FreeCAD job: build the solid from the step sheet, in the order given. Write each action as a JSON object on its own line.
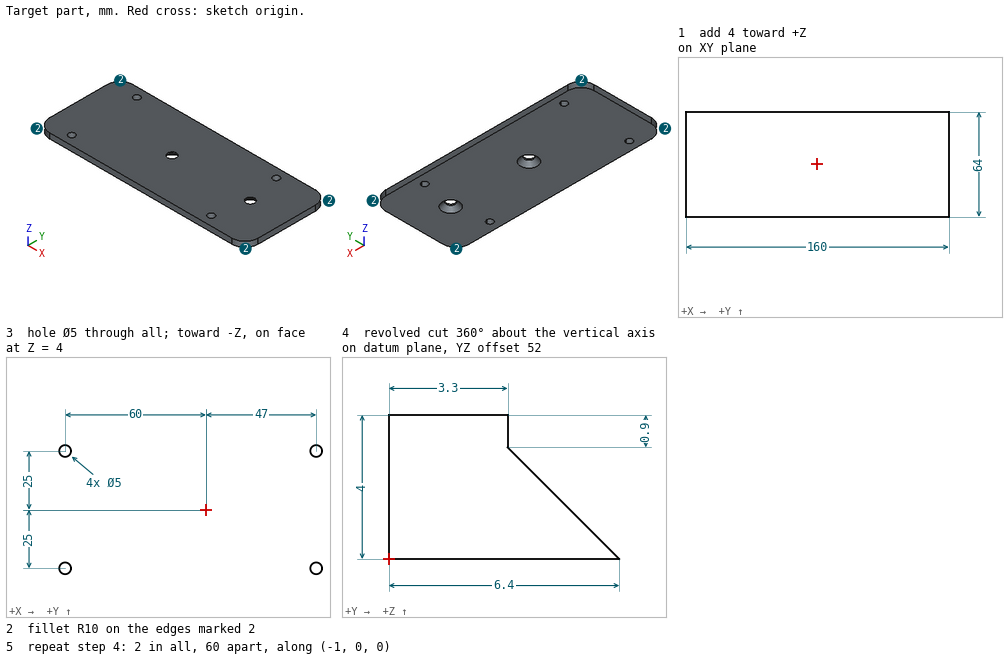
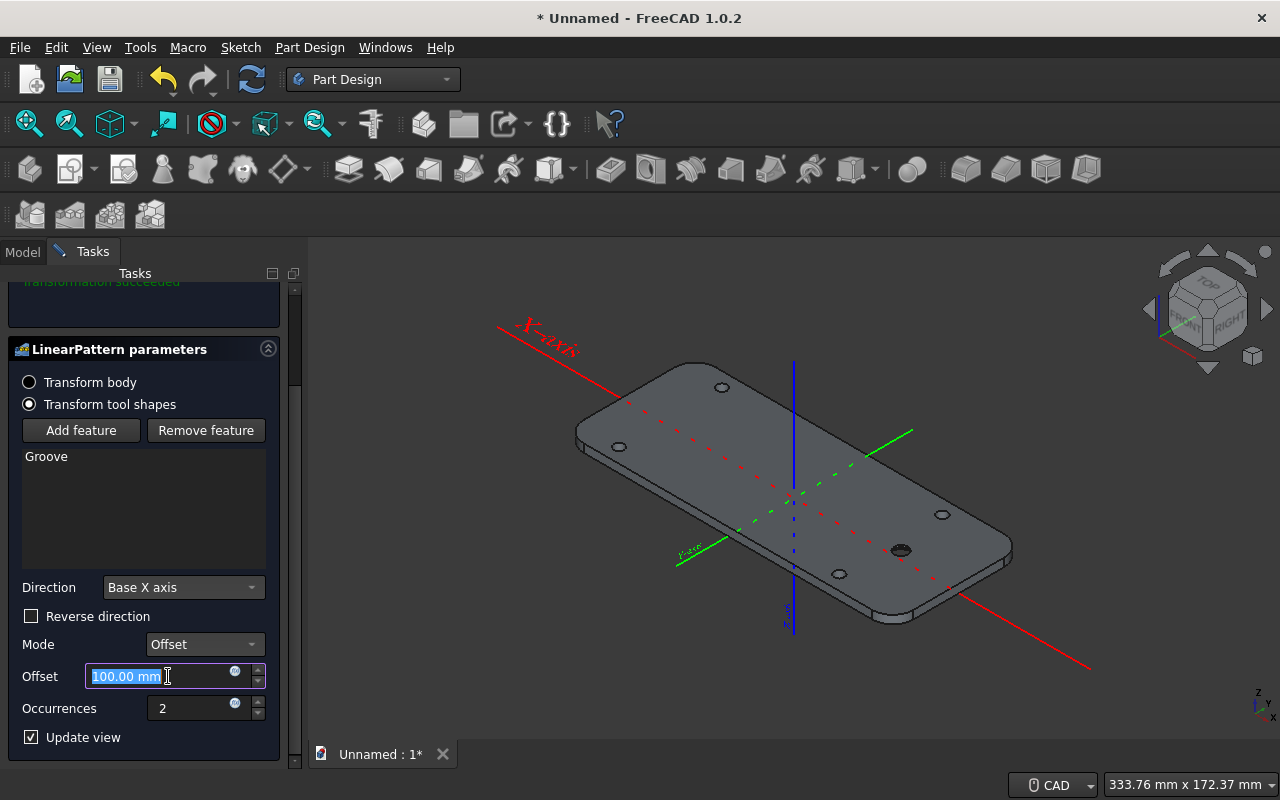
{"action": "type", "text": "60"}
{"action": "key", "text": "Tab"}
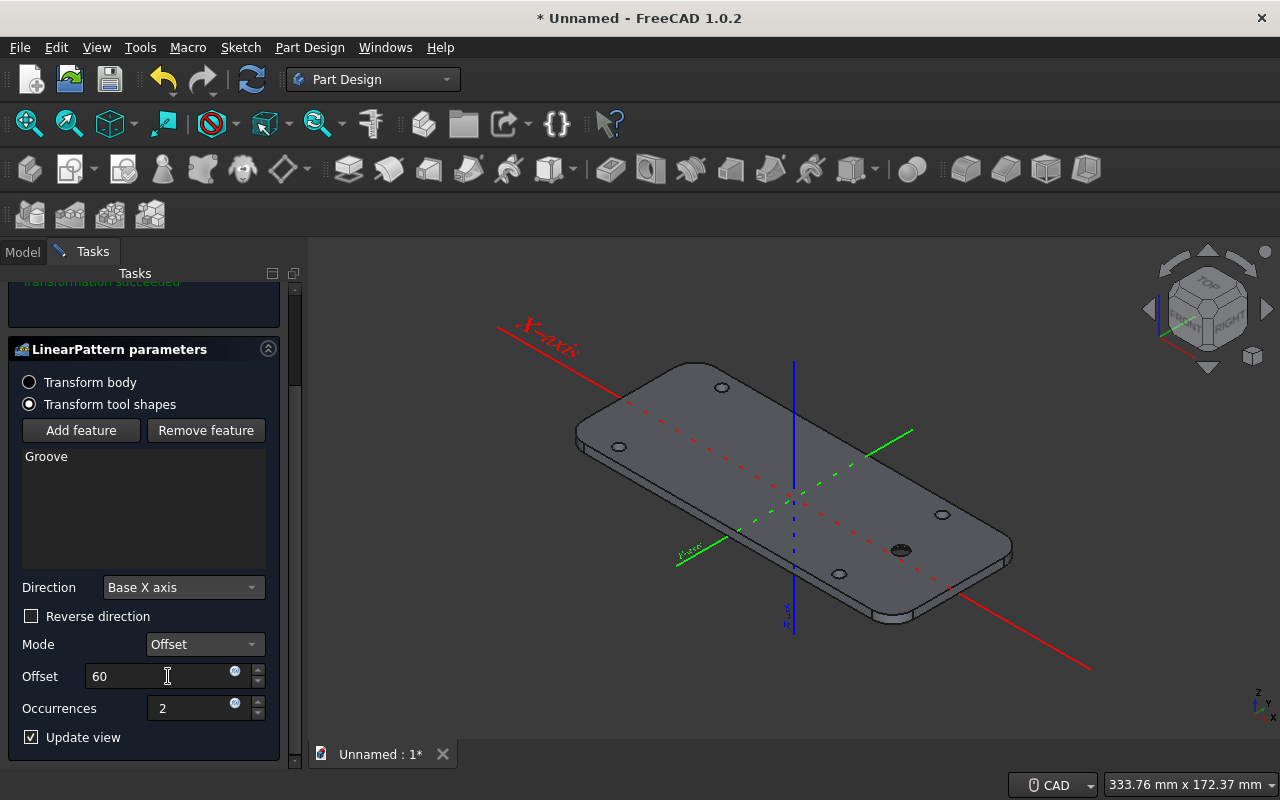
{"action": "triple_click", "coordinate": [198, 708]}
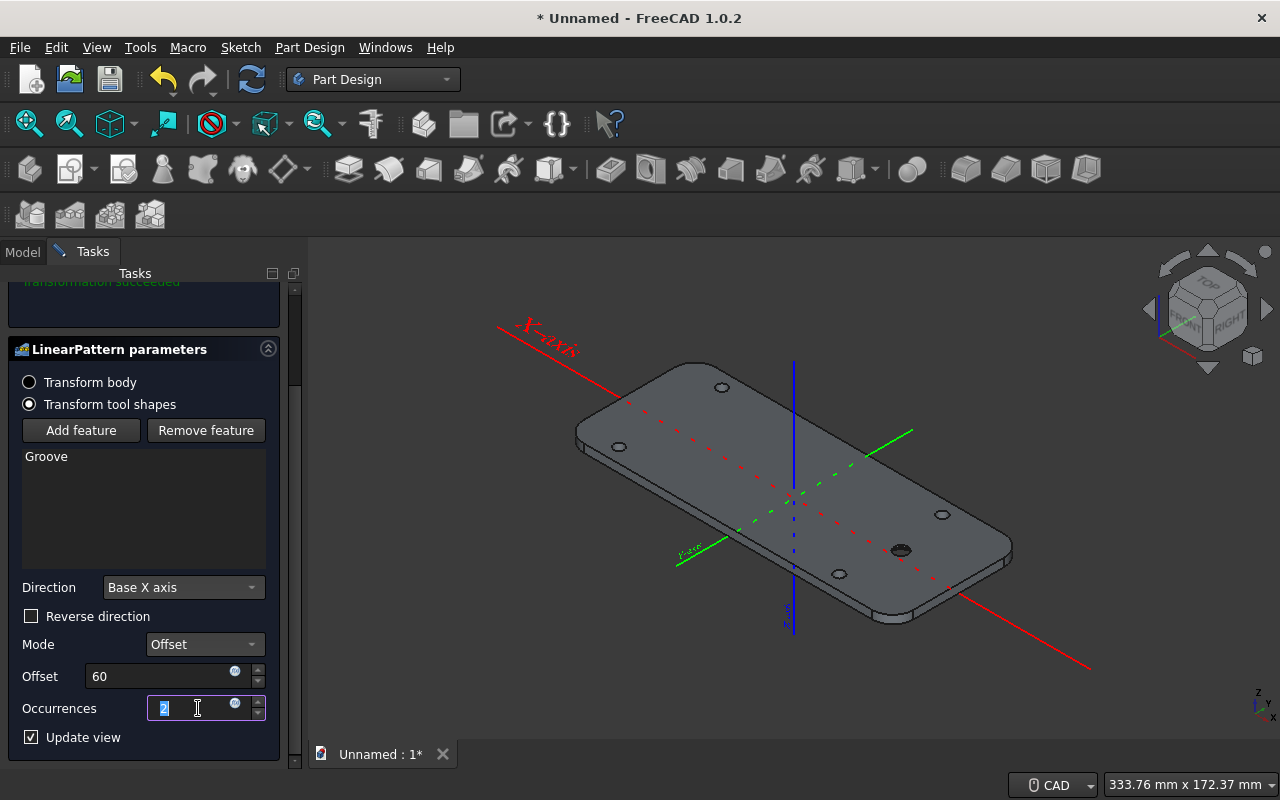
{"action": "type", "text": "2"}
{"action": "key", "text": "Tab"}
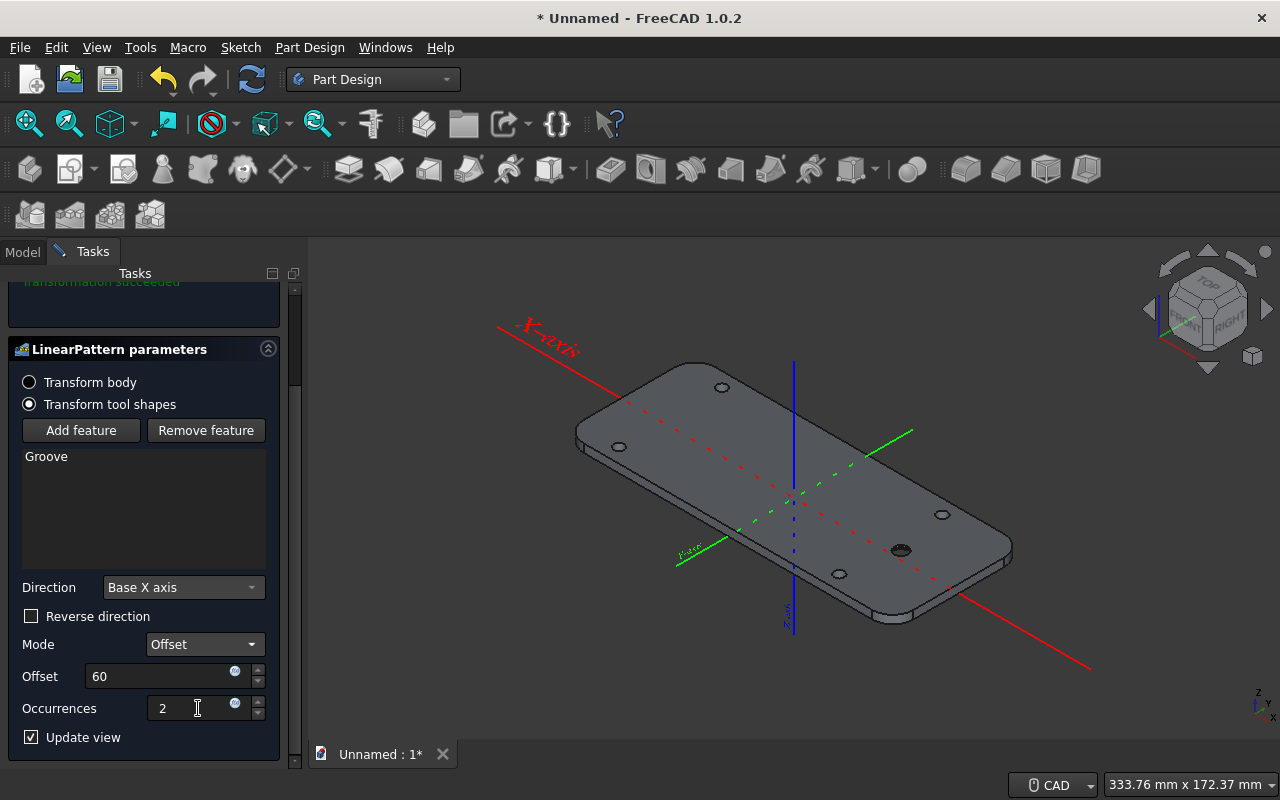
{"action": "left_click", "coordinate": [30, 616]}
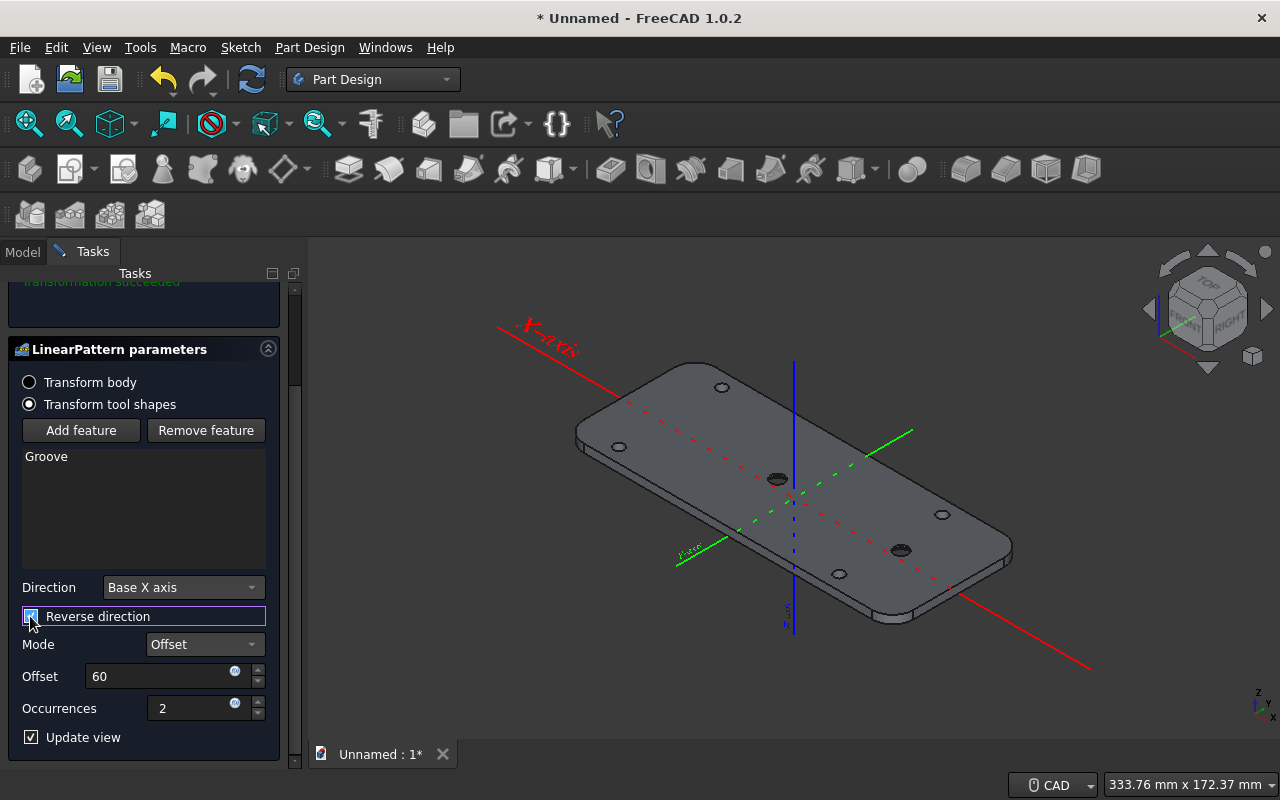
{"action": "scroll", "coordinate": [295, 526], "scroll_direction": "up", "scroll_amount": 3}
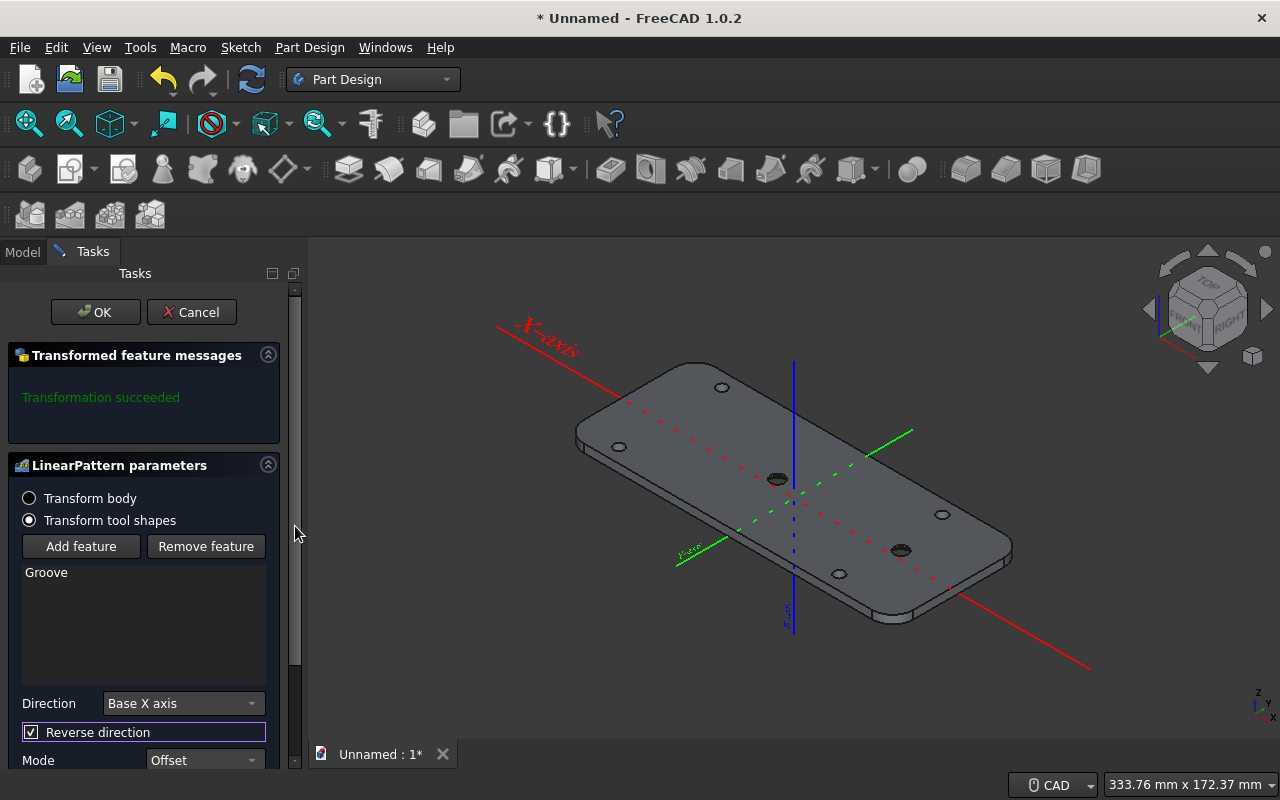
{"action": "left_click", "coordinate": [96, 312]}